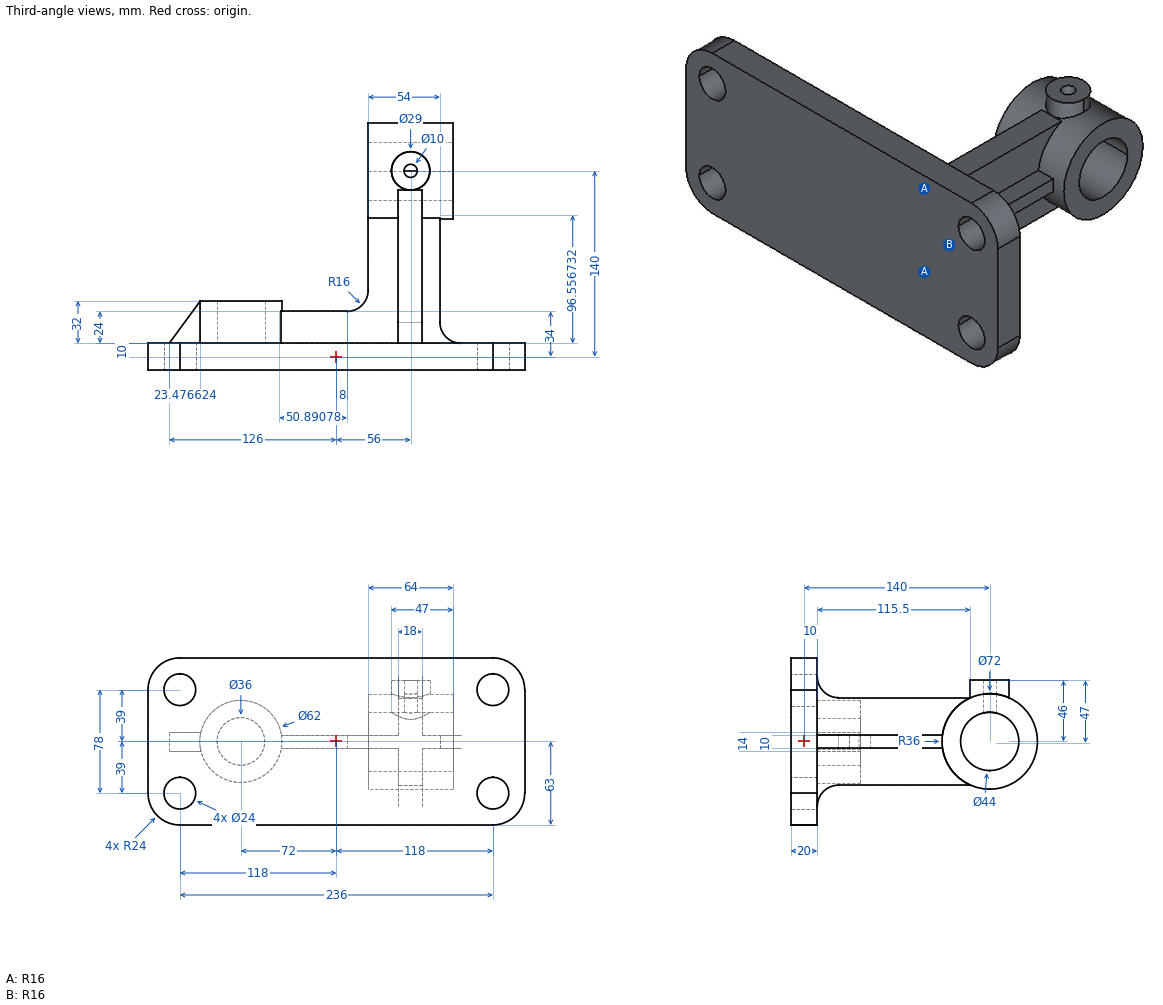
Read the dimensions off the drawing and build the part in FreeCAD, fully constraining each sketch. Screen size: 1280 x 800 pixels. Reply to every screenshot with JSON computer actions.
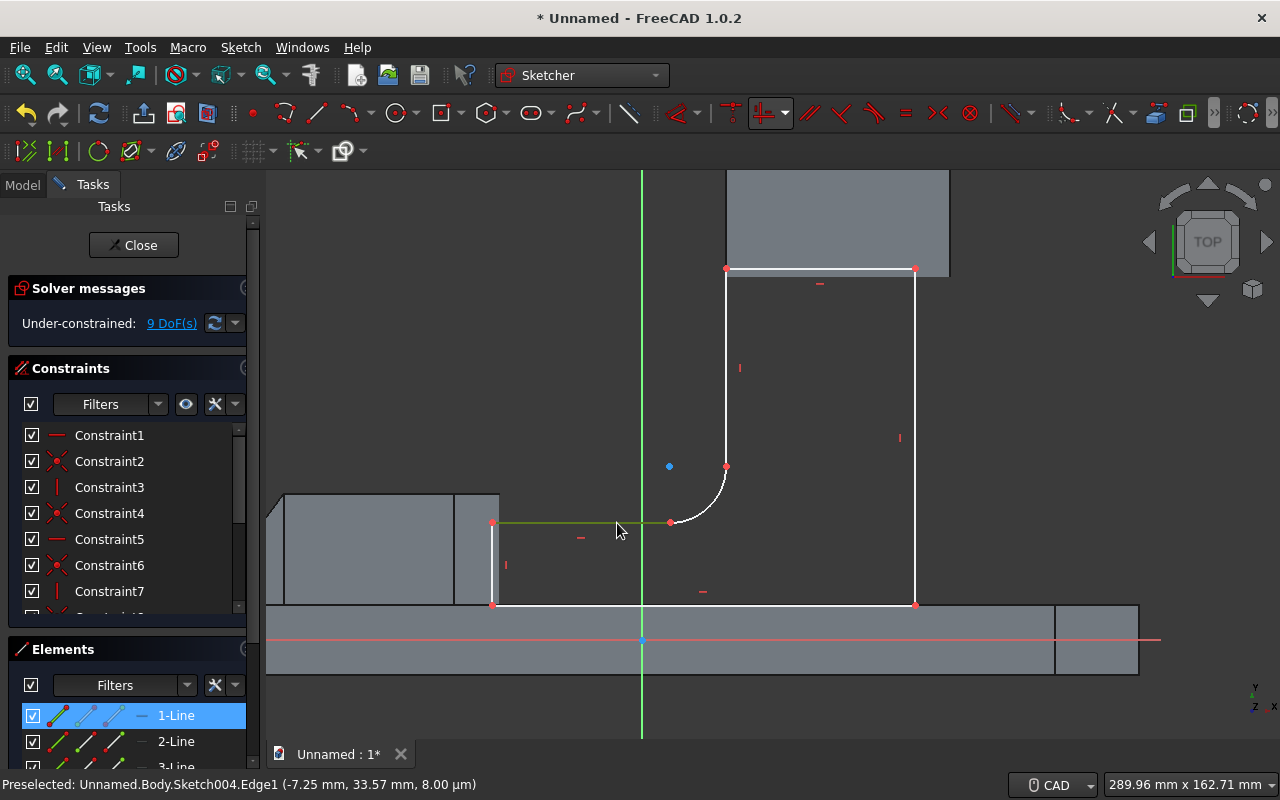
{"action": "left_click", "coordinate": [695, 517]}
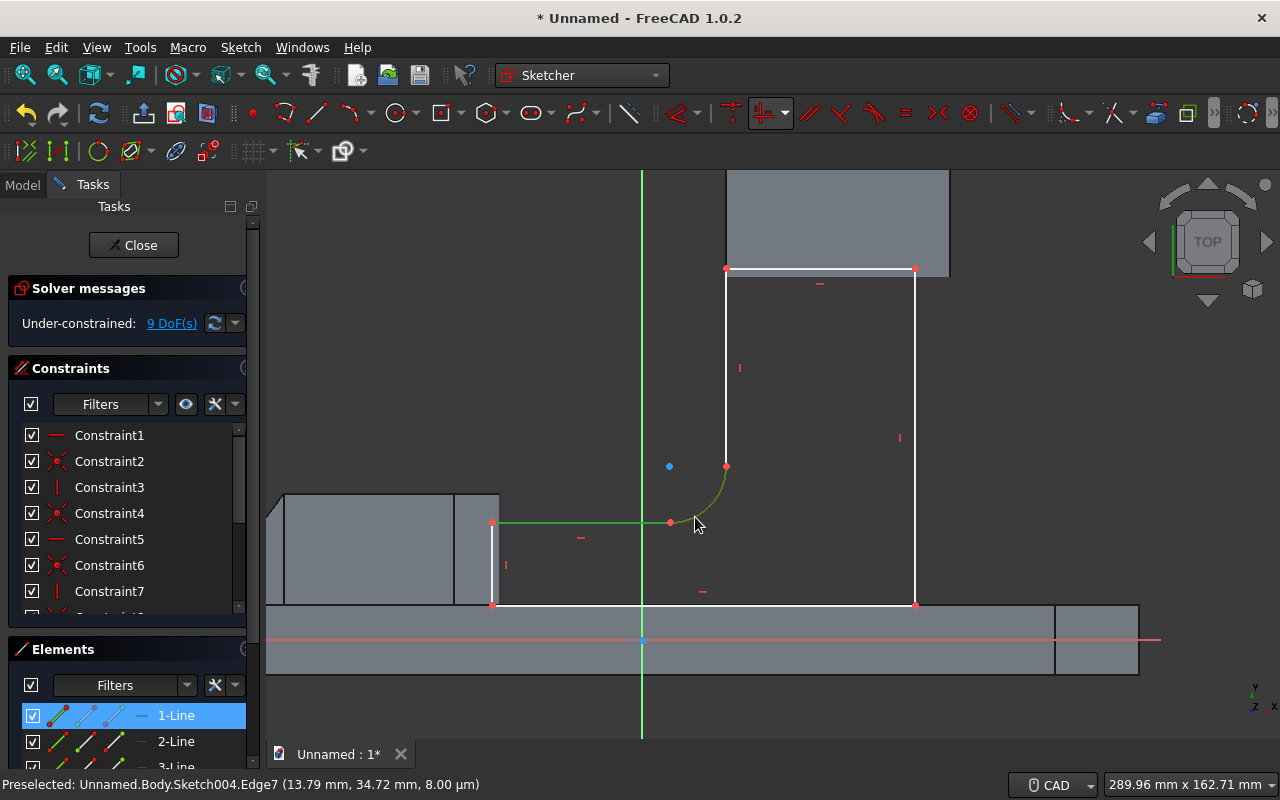
{"action": "left_click", "coordinate": [874, 114]}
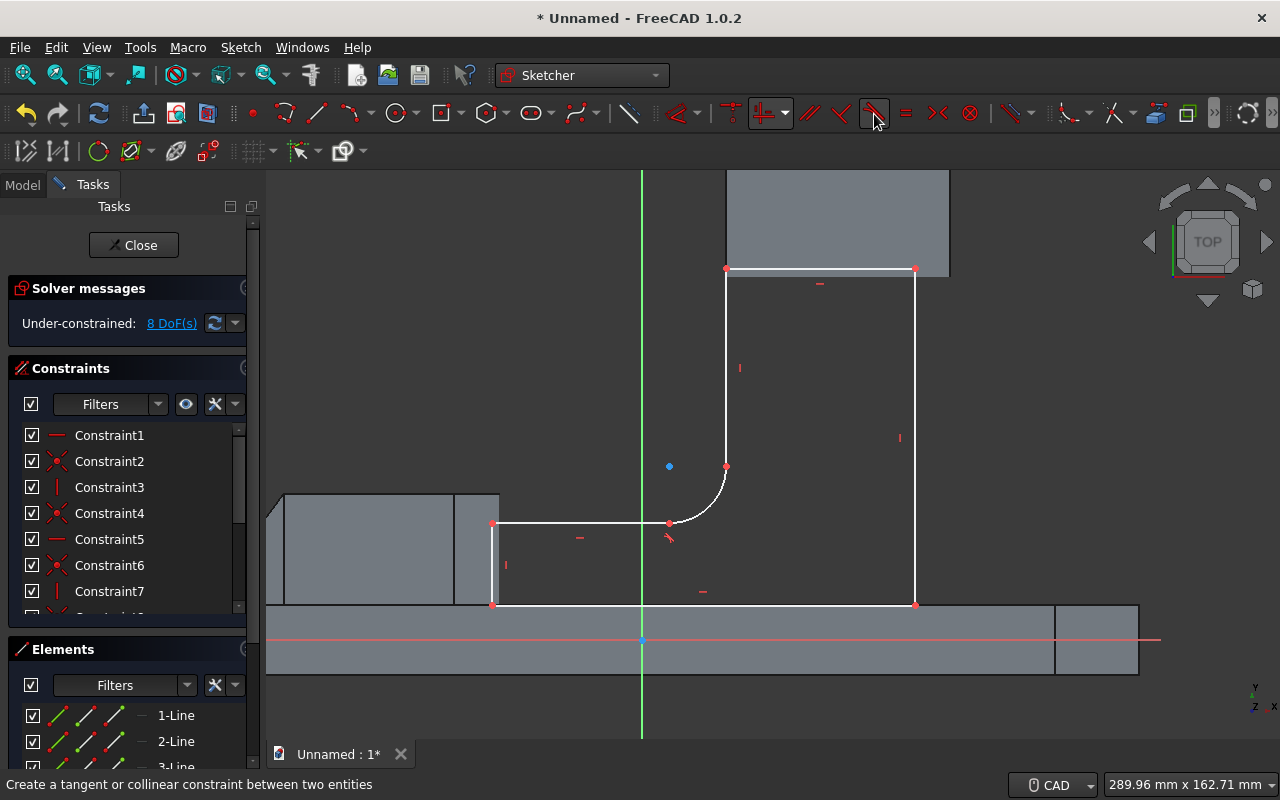
{"action": "left_click", "coordinate": [726, 328]}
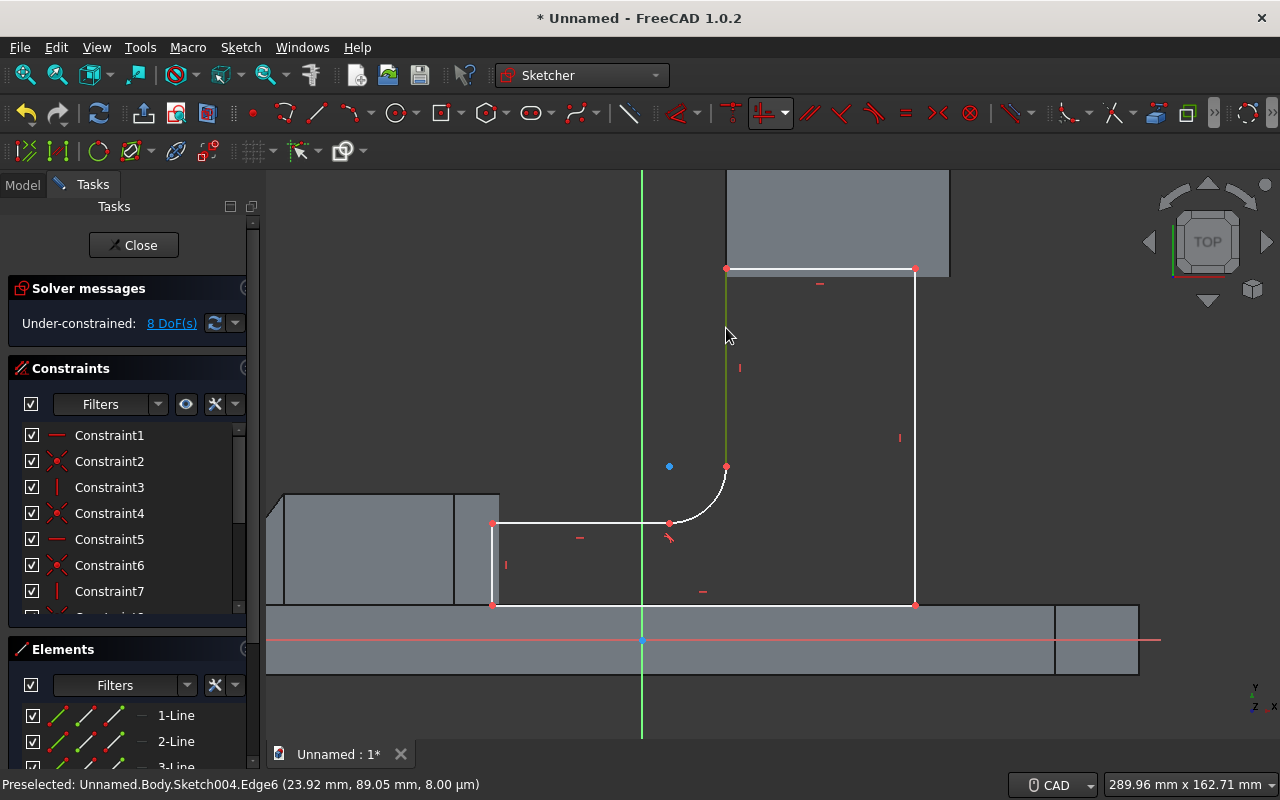
{"action": "left_click", "coordinate": [695, 517]}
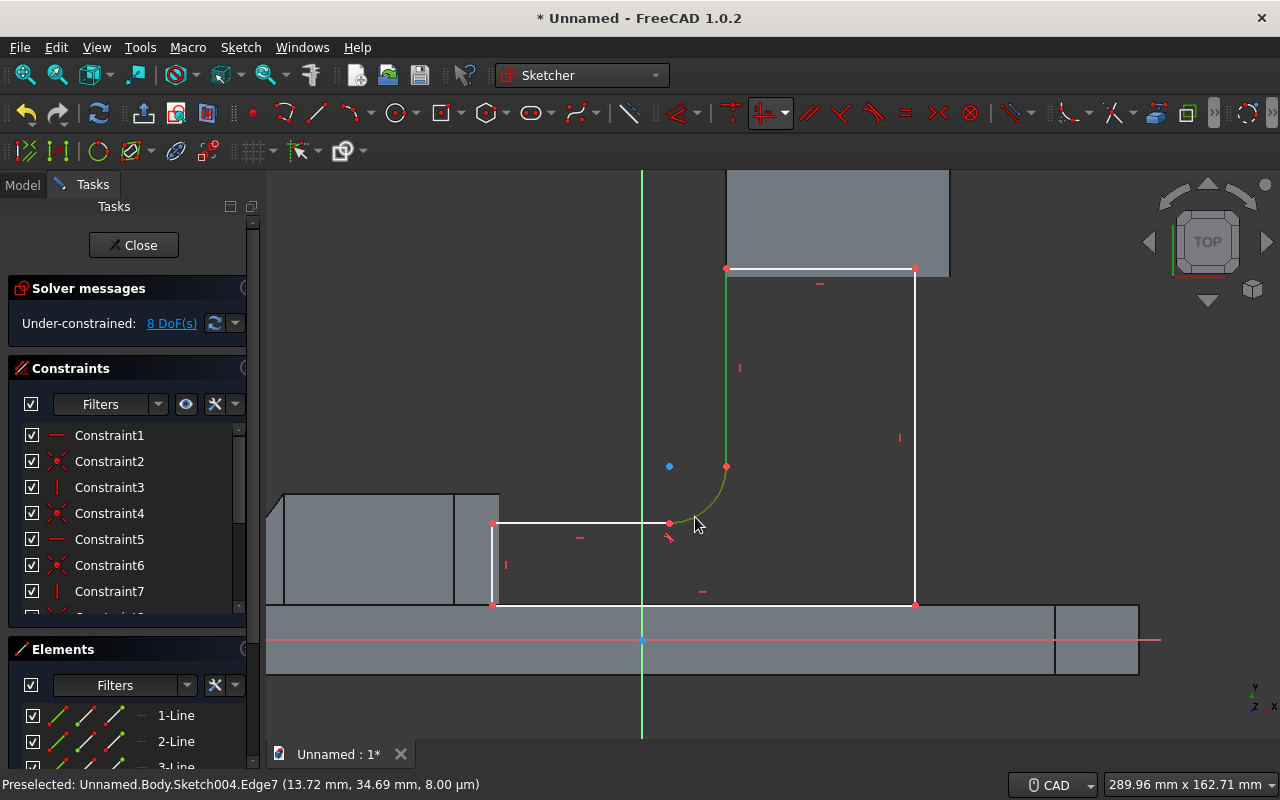
{"action": "left_click", "coordinate": [874, 114]}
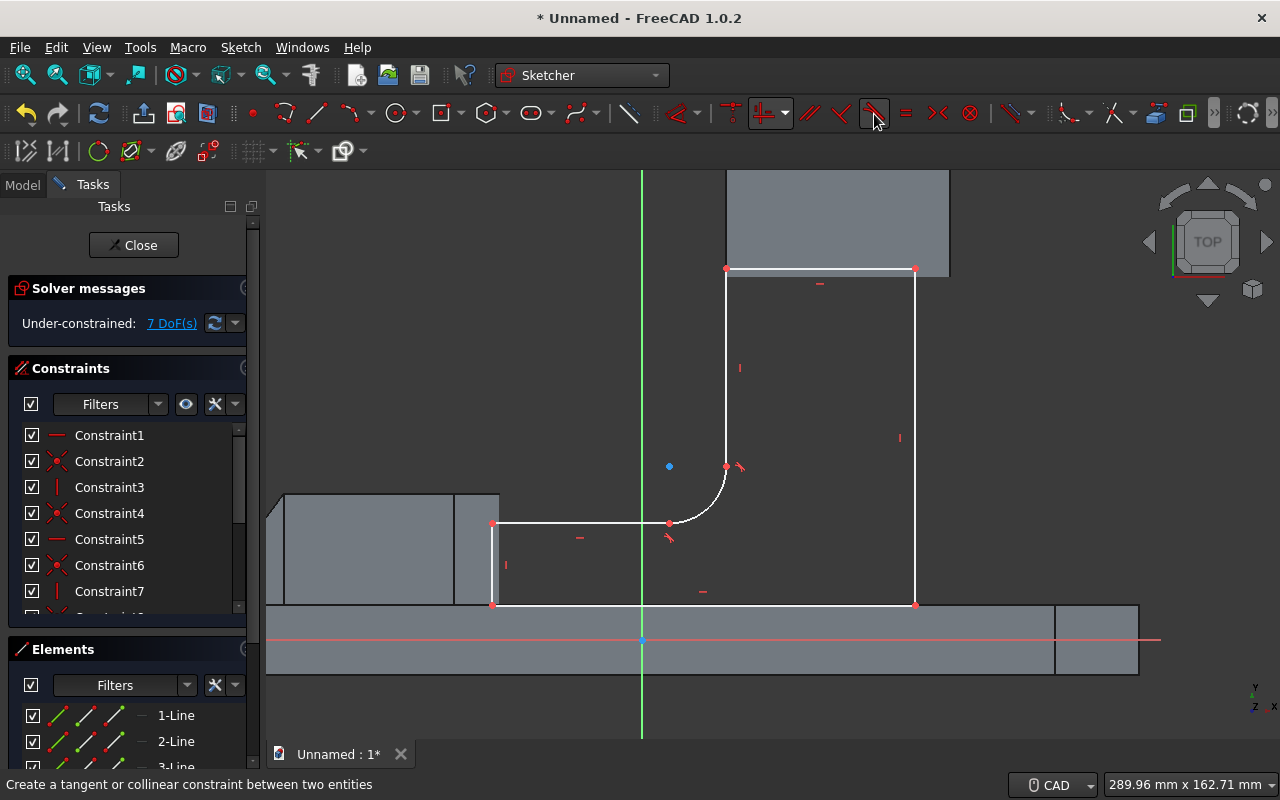
{"action": "left_click", "coordinate": [676, 114]}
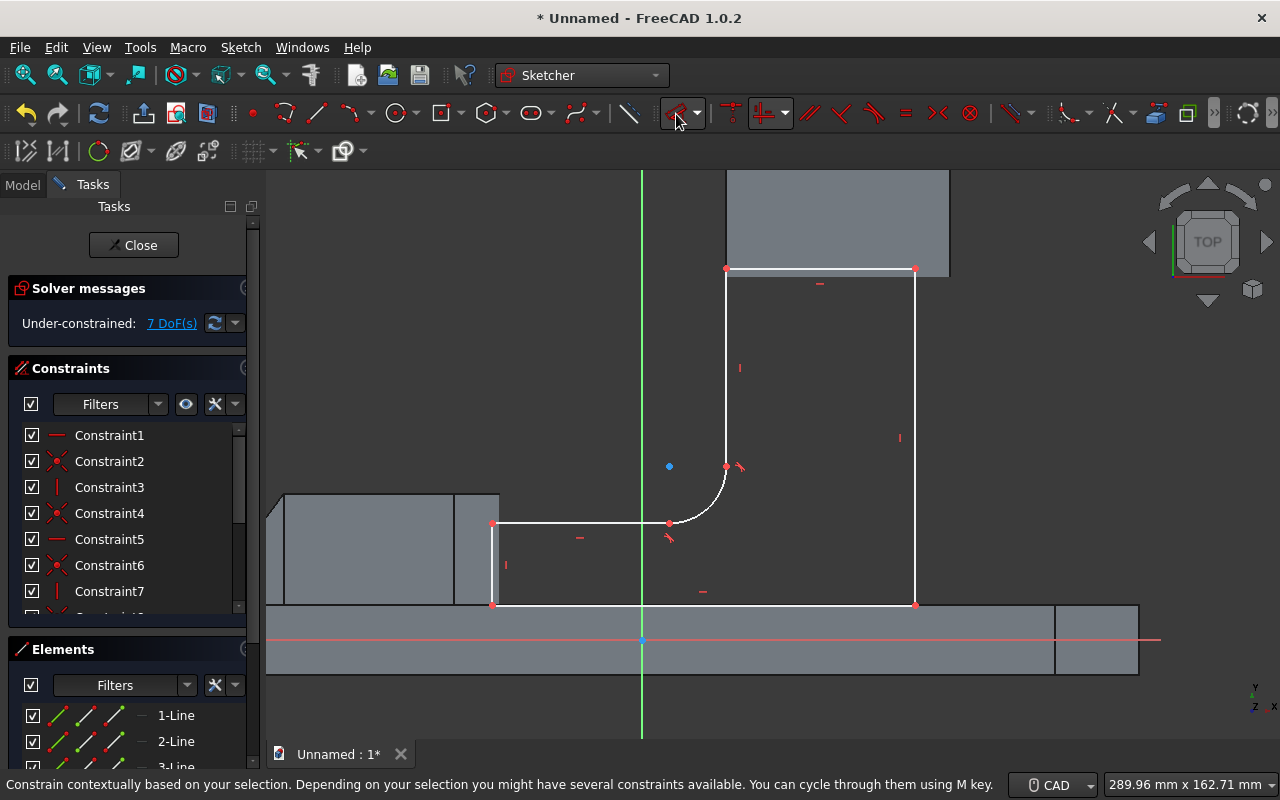
{"action": "left_click", "coordinate": [695, 517]}
{"action": "left_click", "coordinate": [709, 546]}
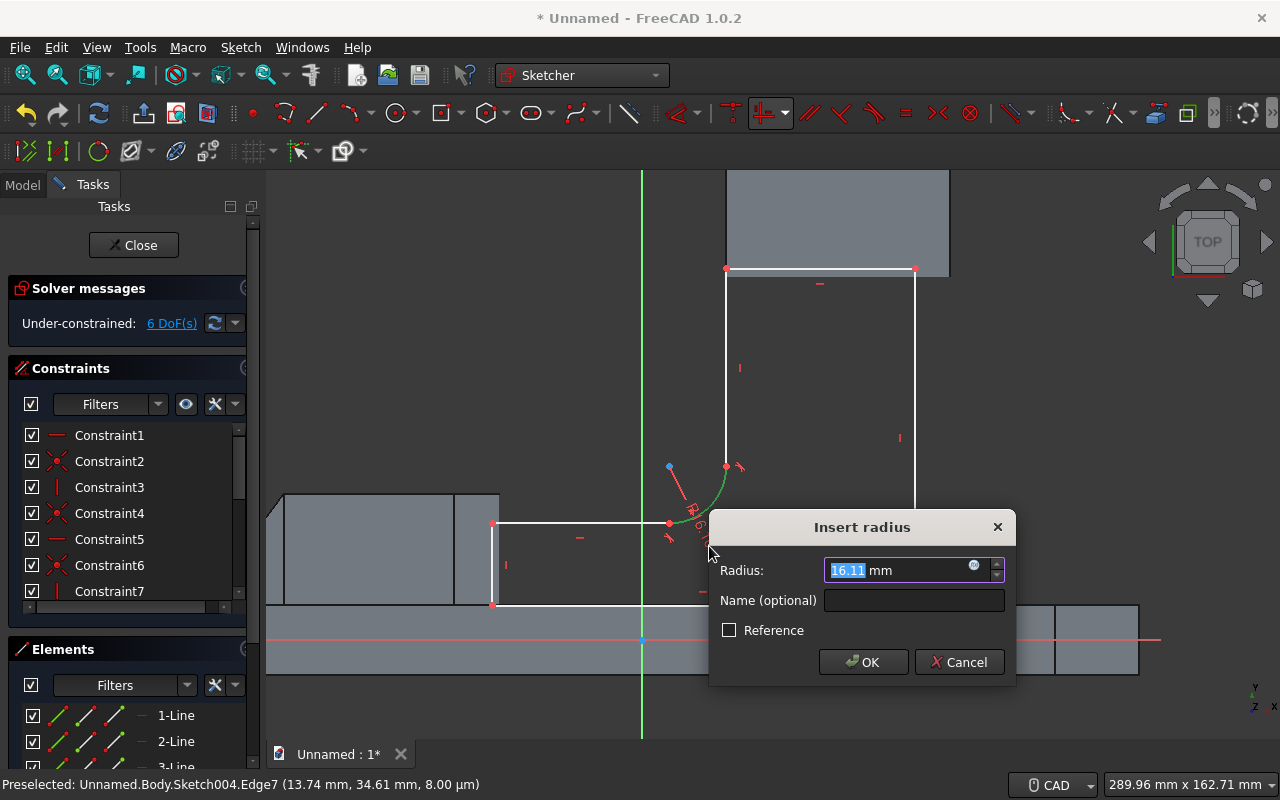
{"action": "type", "text": "16"}
{"action": "key", "text": "Return"}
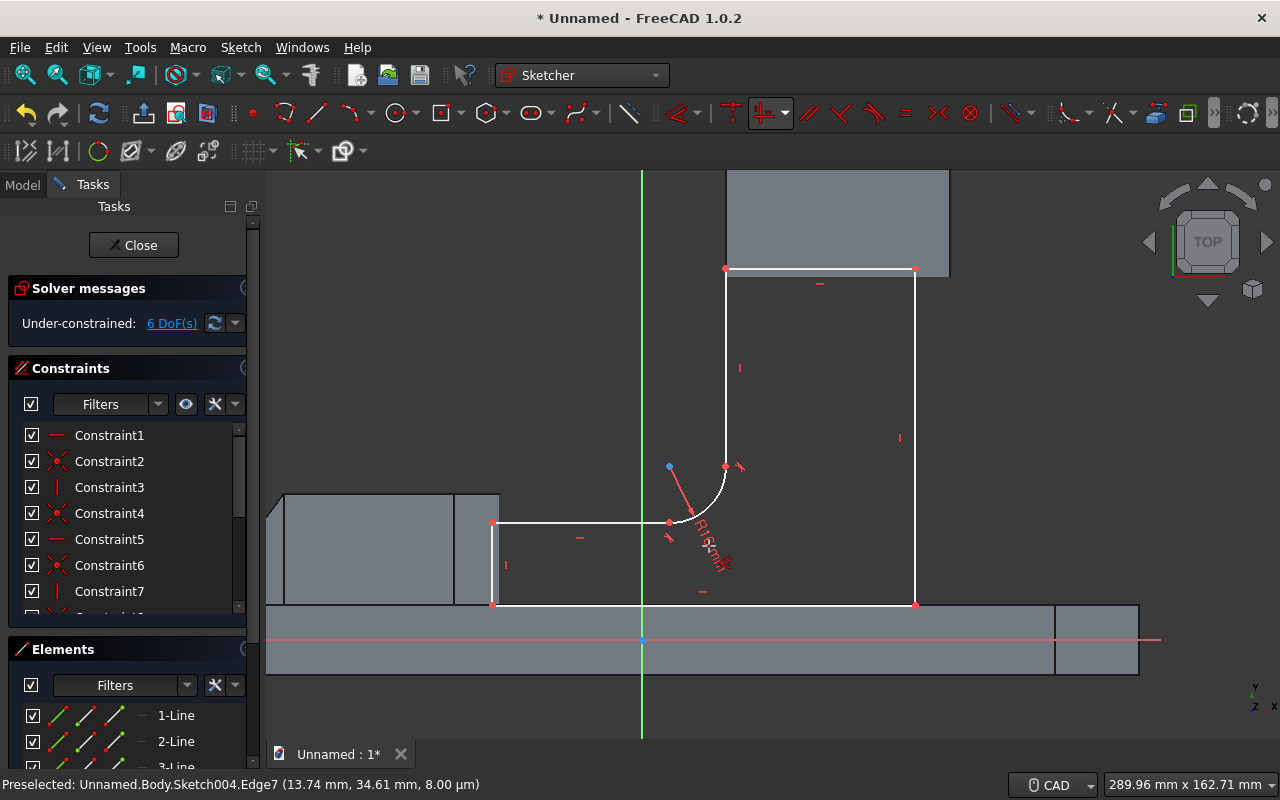
{"action": "left_click", "coordinate": [492, 548]}
{"action": "left_click", "coordinate": [458, 564]}